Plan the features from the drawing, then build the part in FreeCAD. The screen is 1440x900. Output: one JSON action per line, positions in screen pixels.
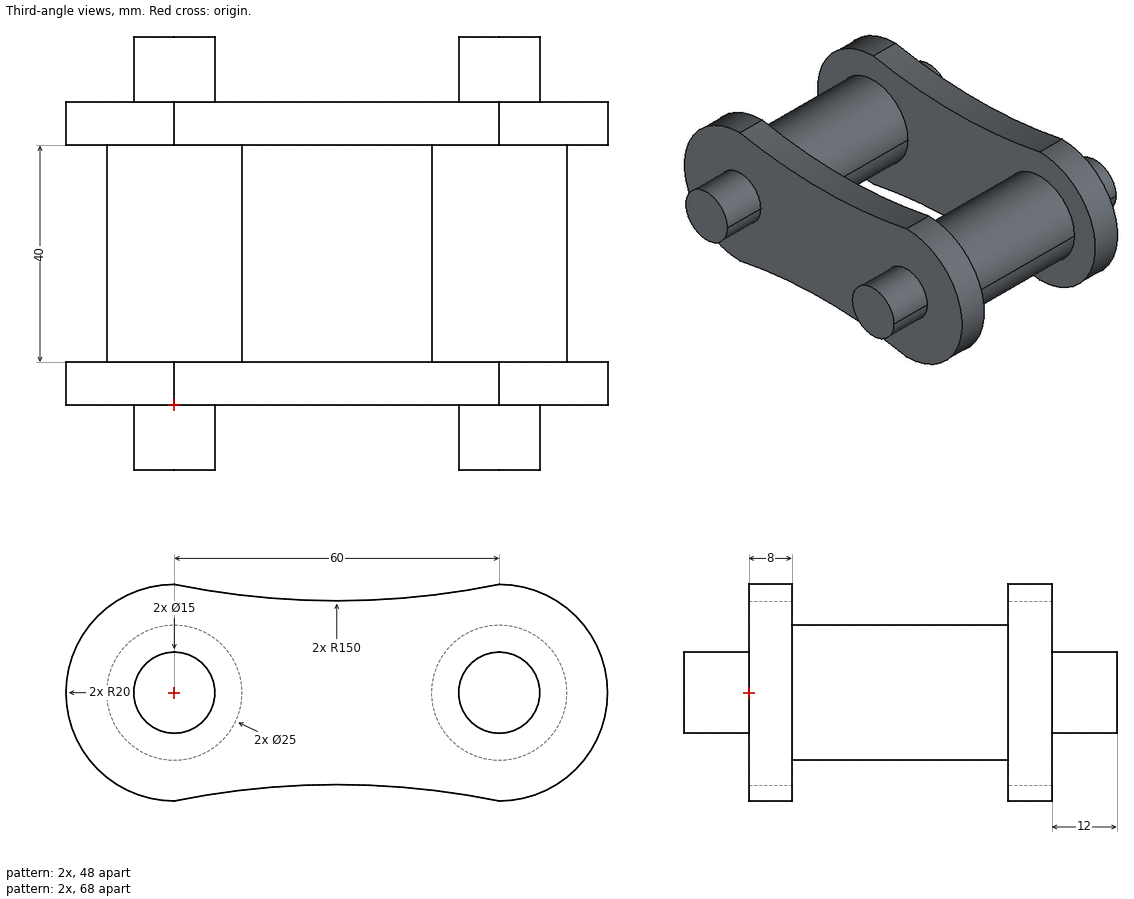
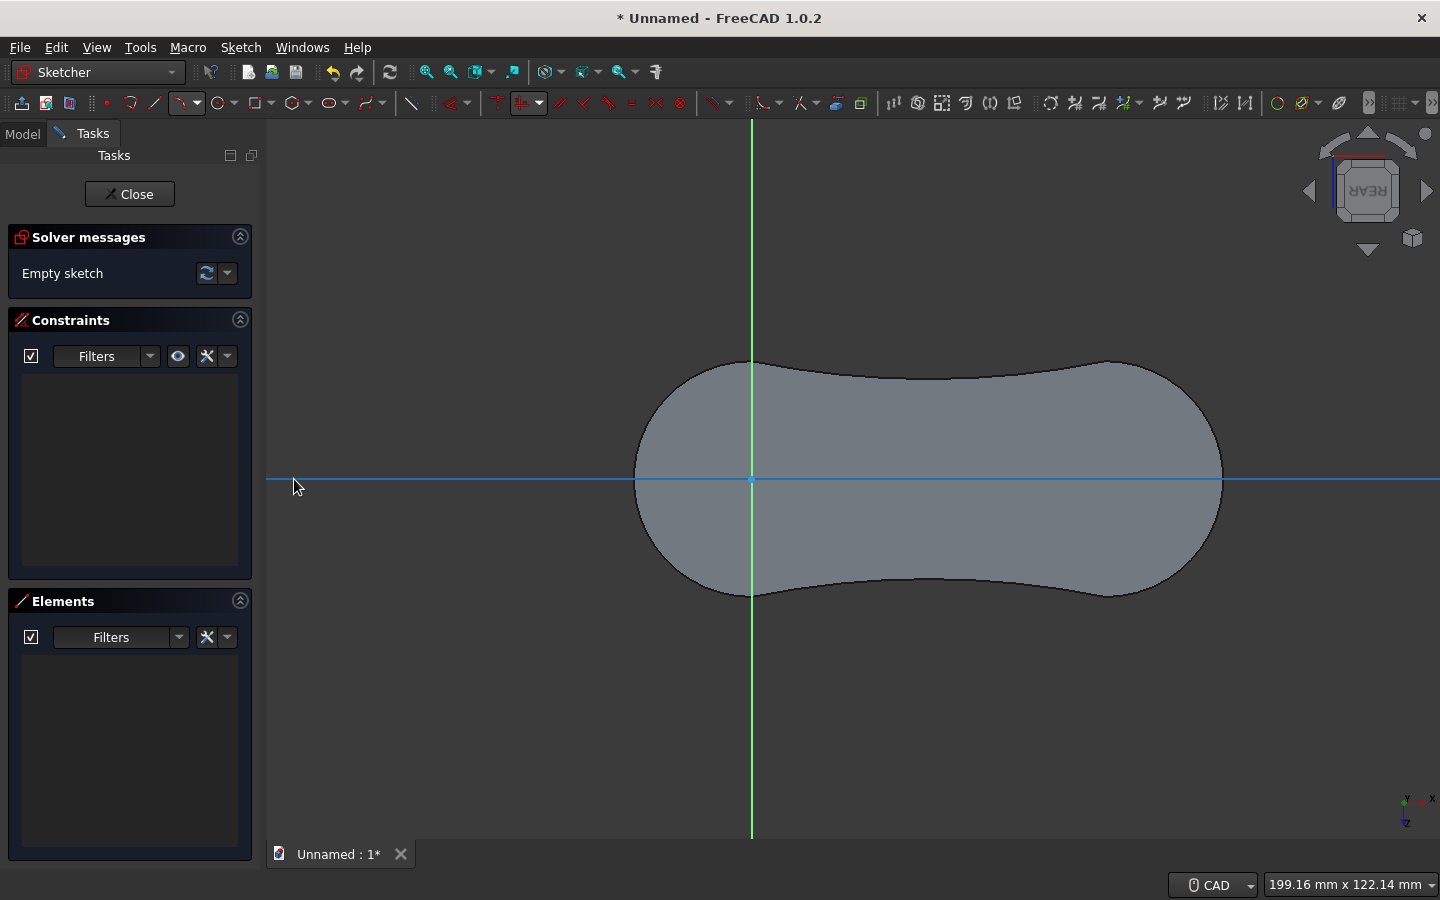
{"action": "scroll", "coordinate": [1221, 479], "scroll_direction": "up", "scroll_amount": 2}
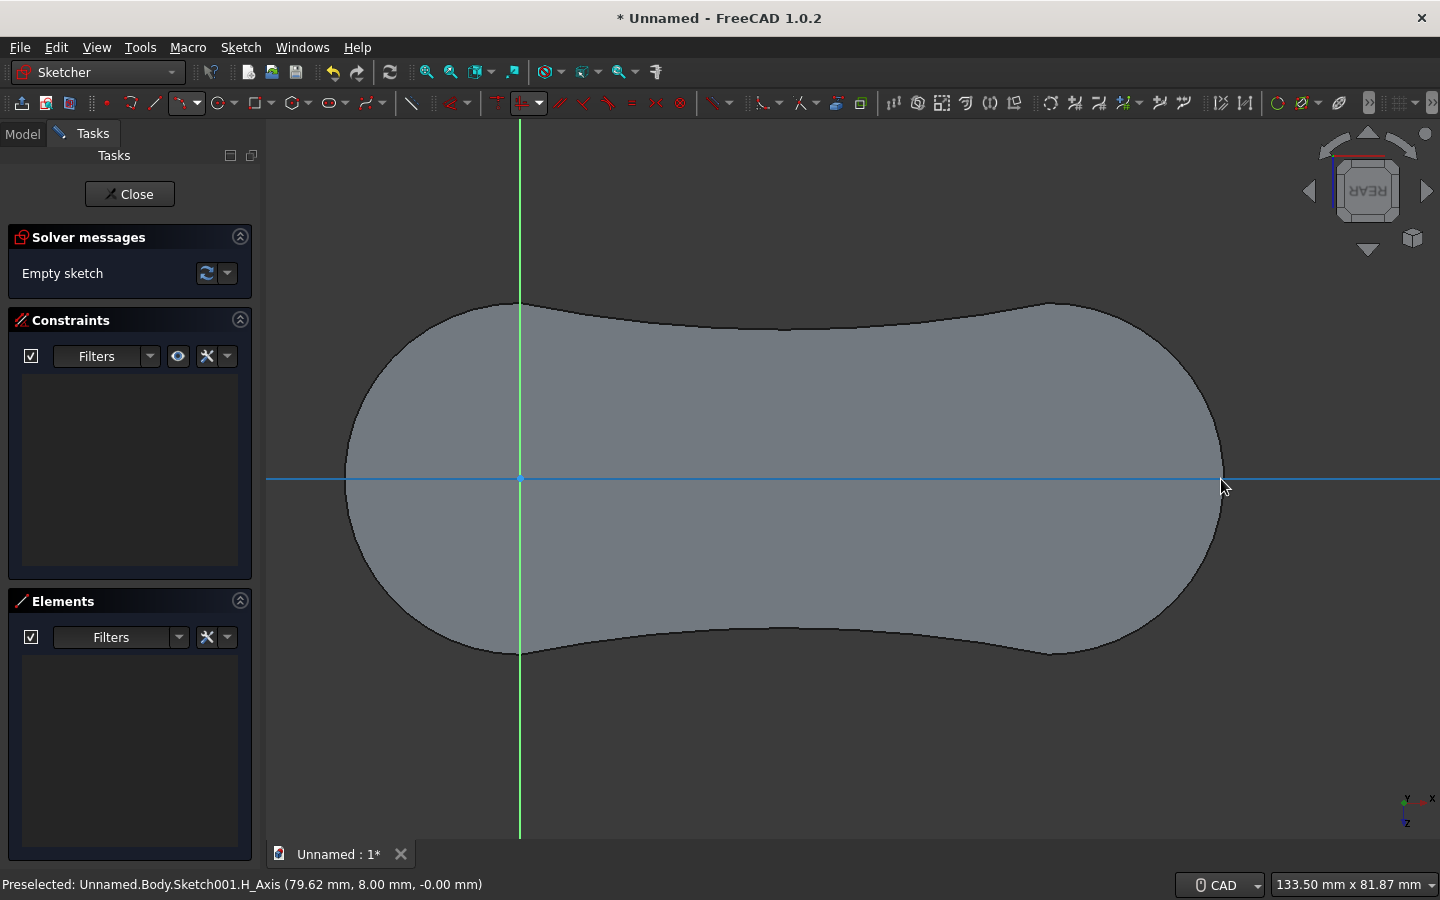
{"action": "left_click", "coordinate": [218, 104]}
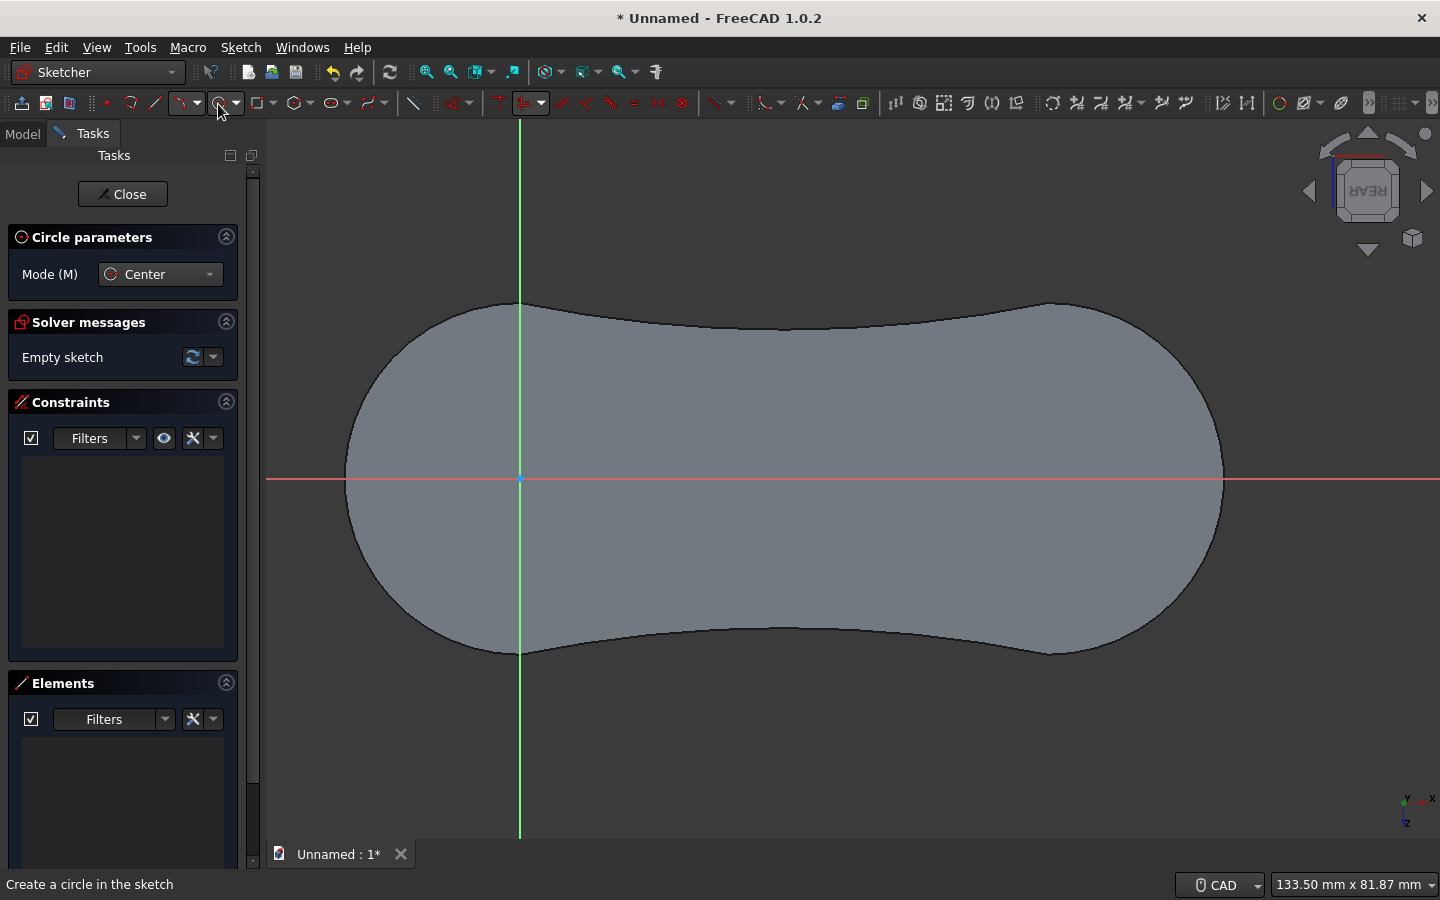
{"action": "left_click", "coordinate": [520, 479]}
{"action": "mouse_move", "coordinate": [598, 401]}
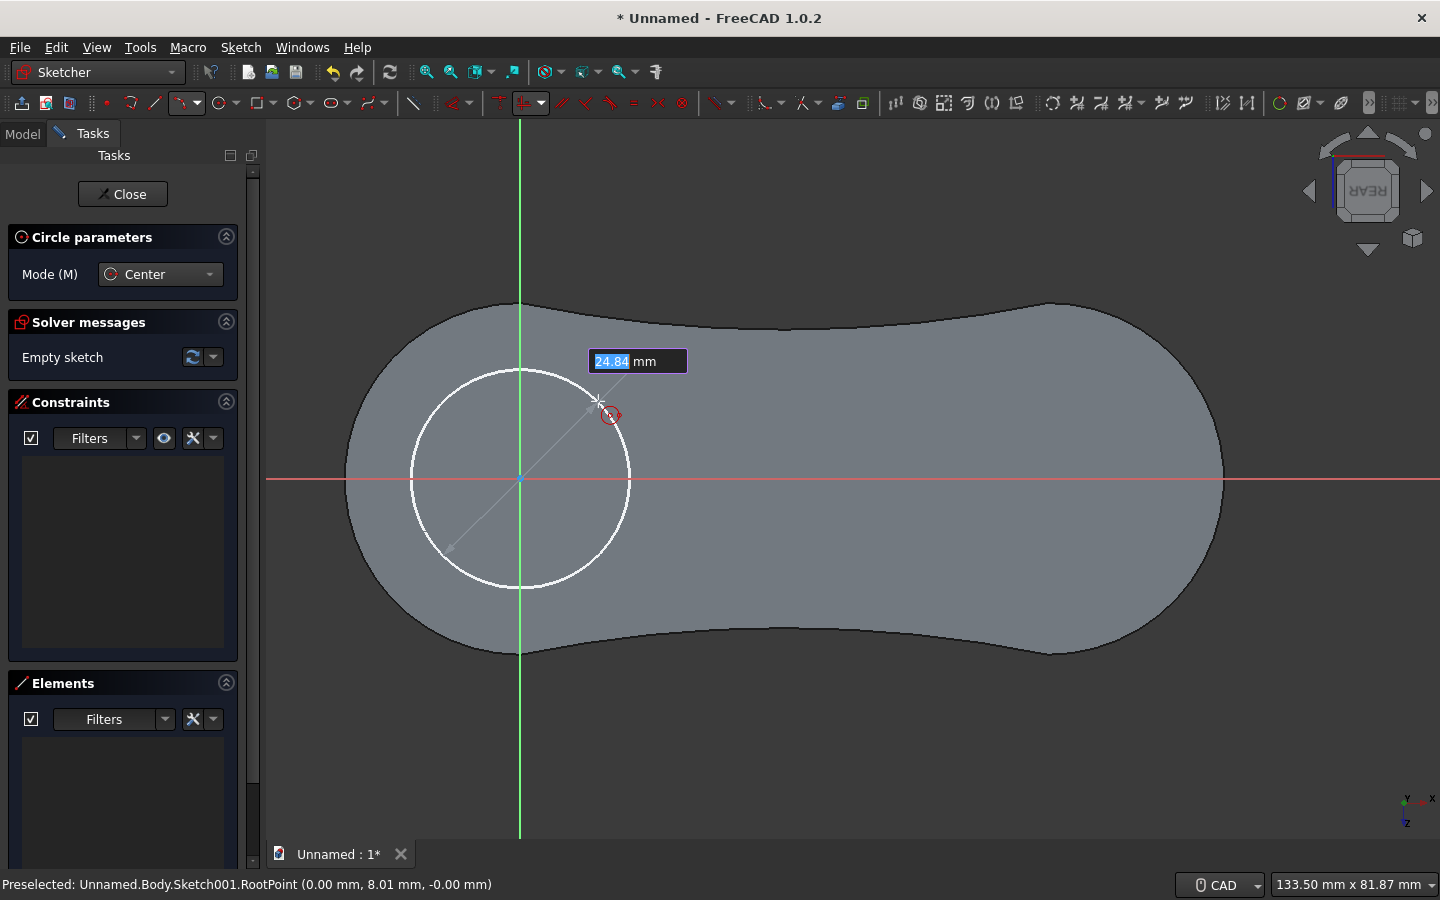
{"action": "type", "text": "25"}
{"action": "key", "text": "Return"}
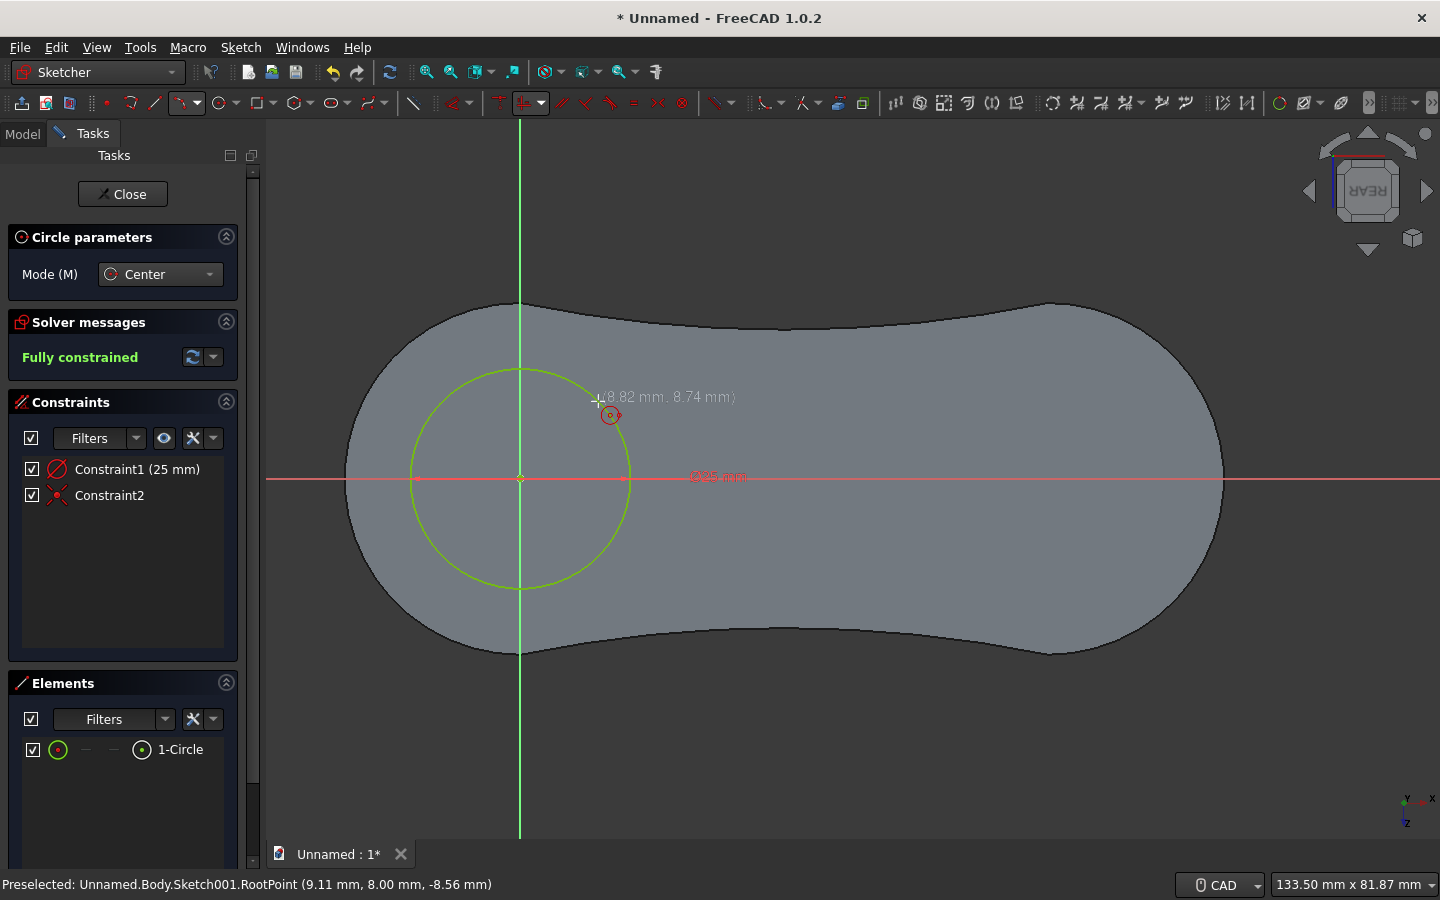
{"action": "left_click", "coordinate": [1048, 479]}
{"action": "mouse_move", "coordinate": [1126, 401]}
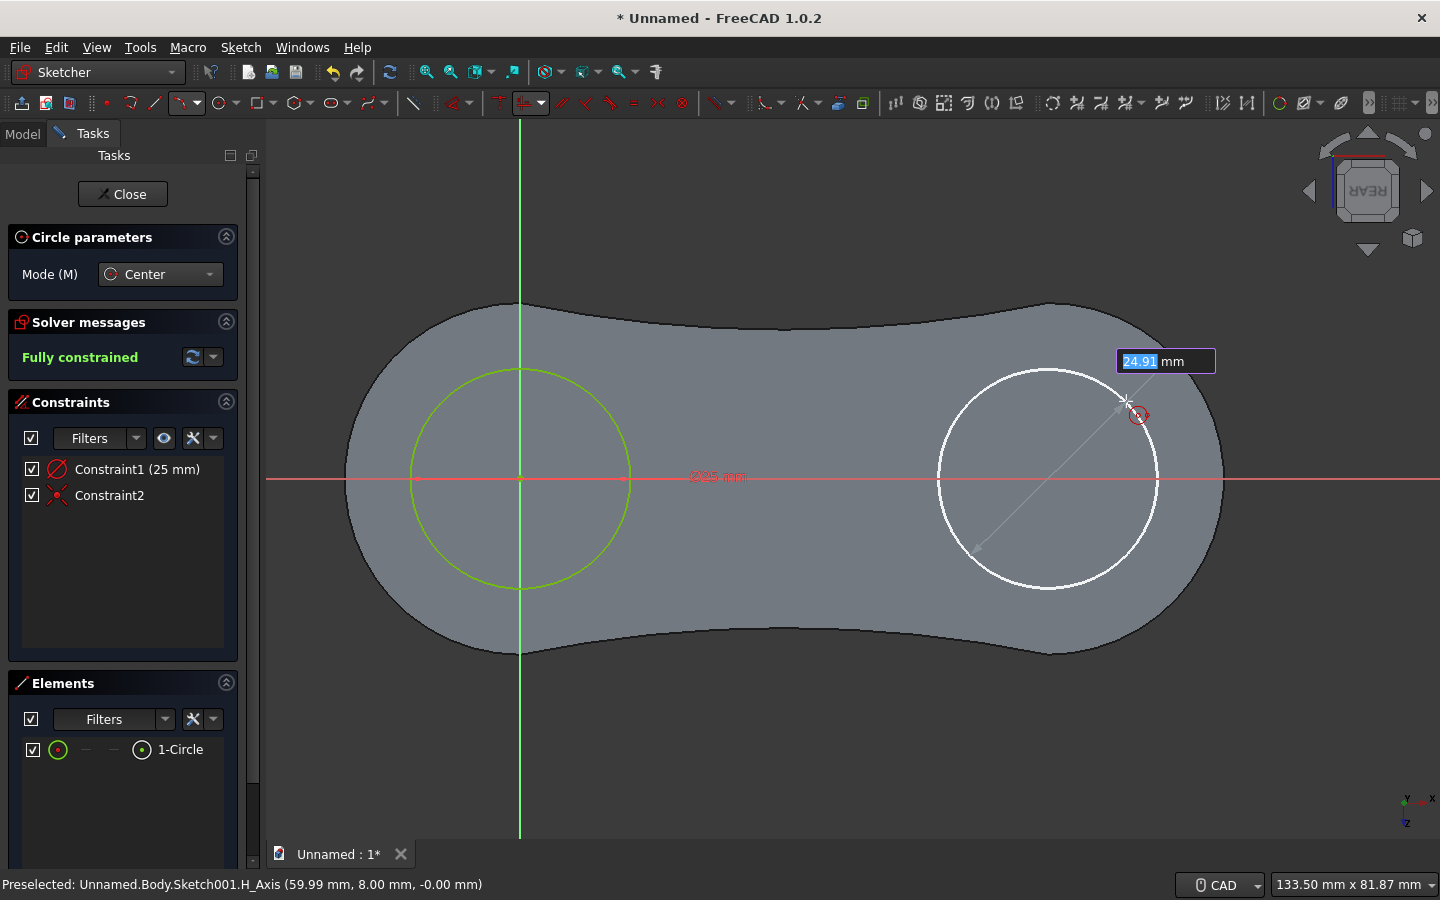
{"action": "type", "text": "25"}
{"action": "key", "text": "Return"}
{"action": "key", "text": "Escape"}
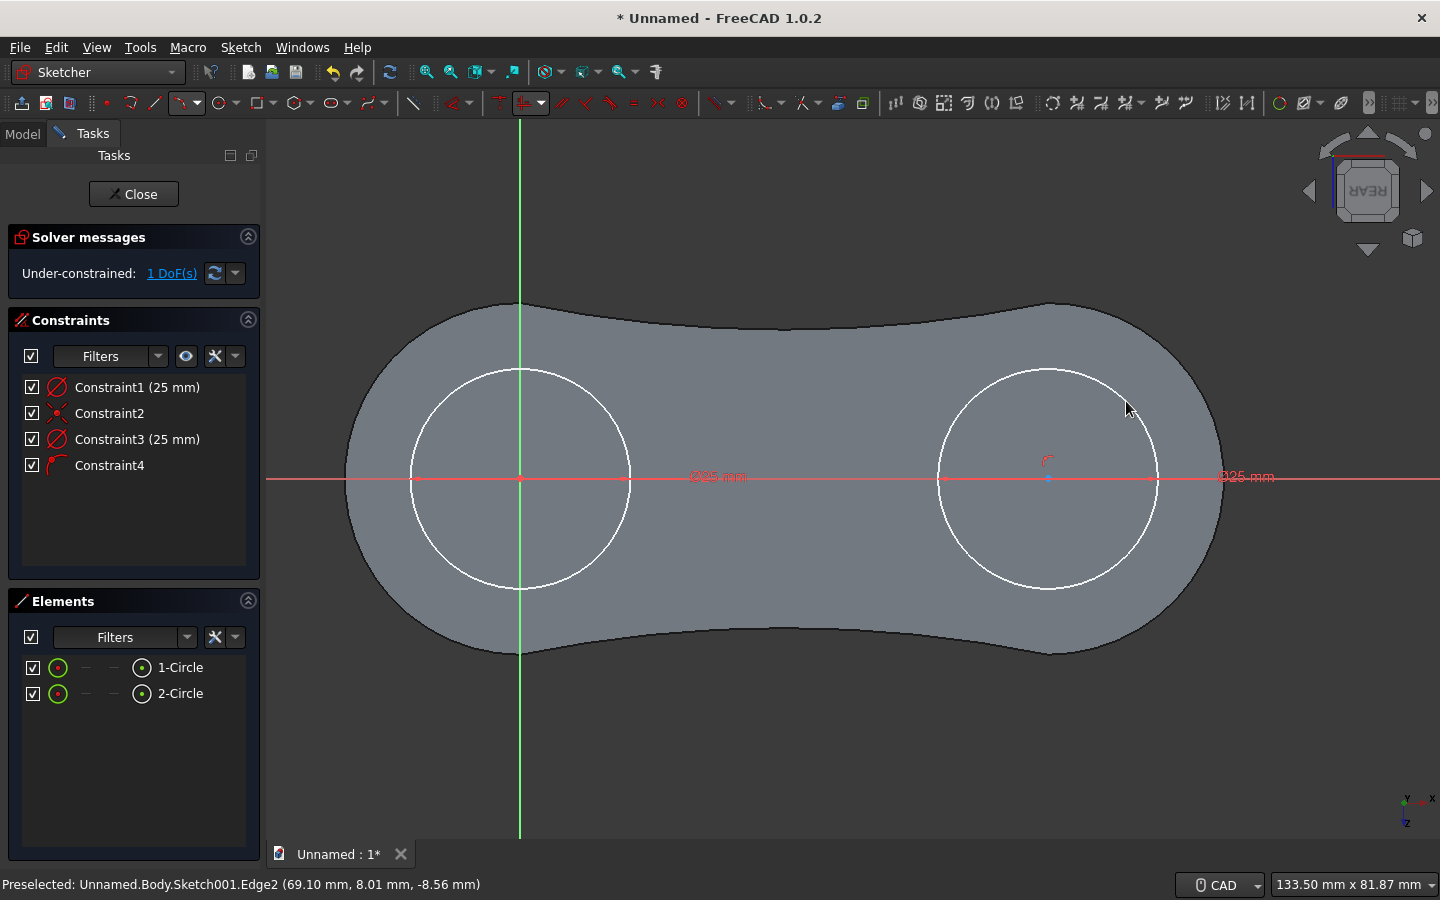
{"action": "left_click", "coordinate": [452, 104]}